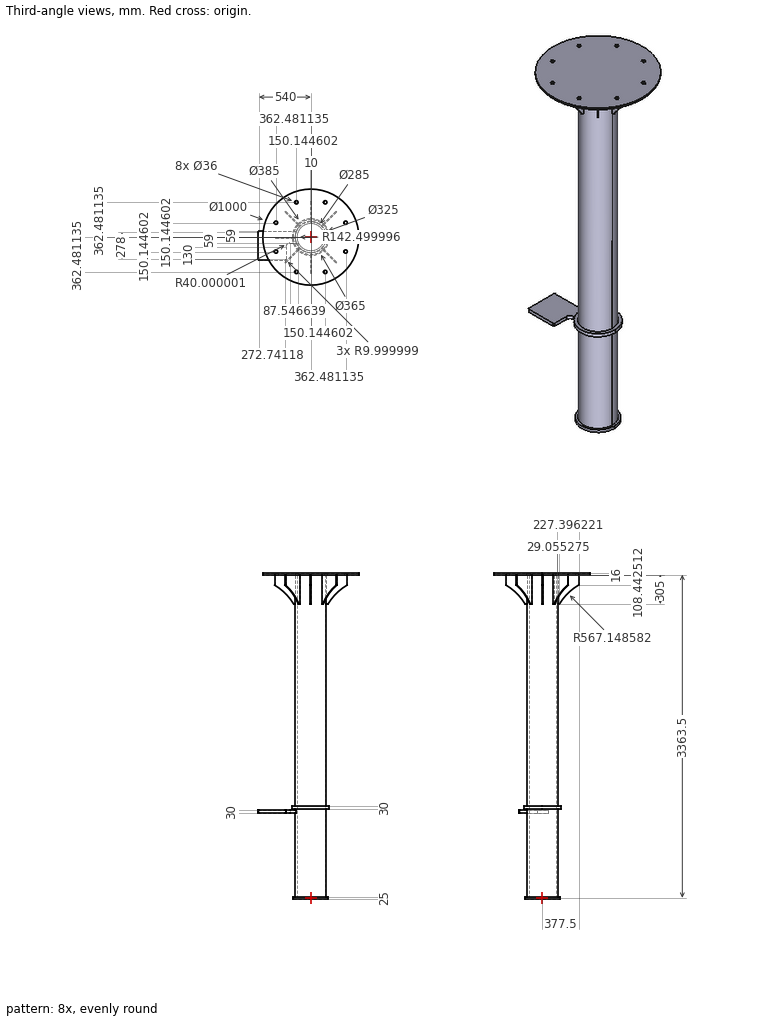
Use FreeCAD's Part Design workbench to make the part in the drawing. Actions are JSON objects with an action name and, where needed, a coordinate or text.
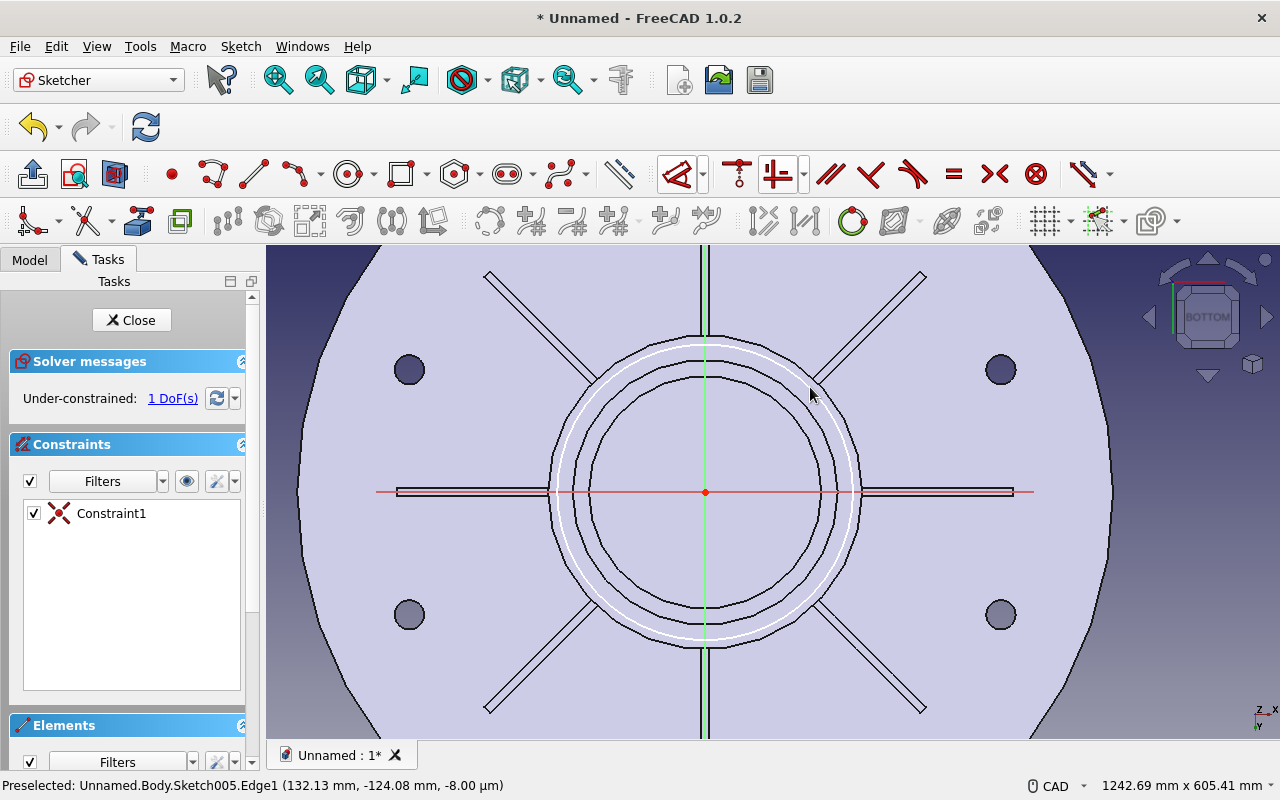
{"action": "left_click", "coordinate": [809, 387]}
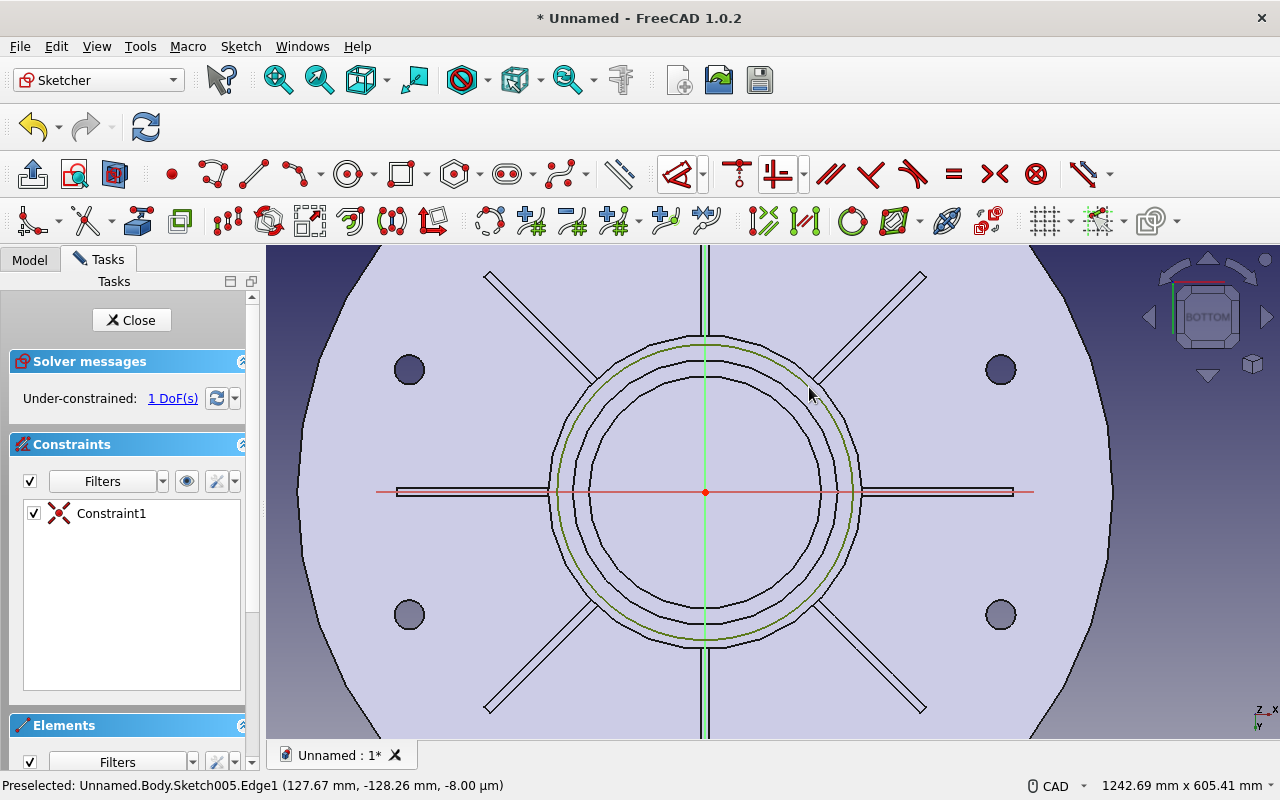
{"action": "left_click", "coordinate": [702, 174]}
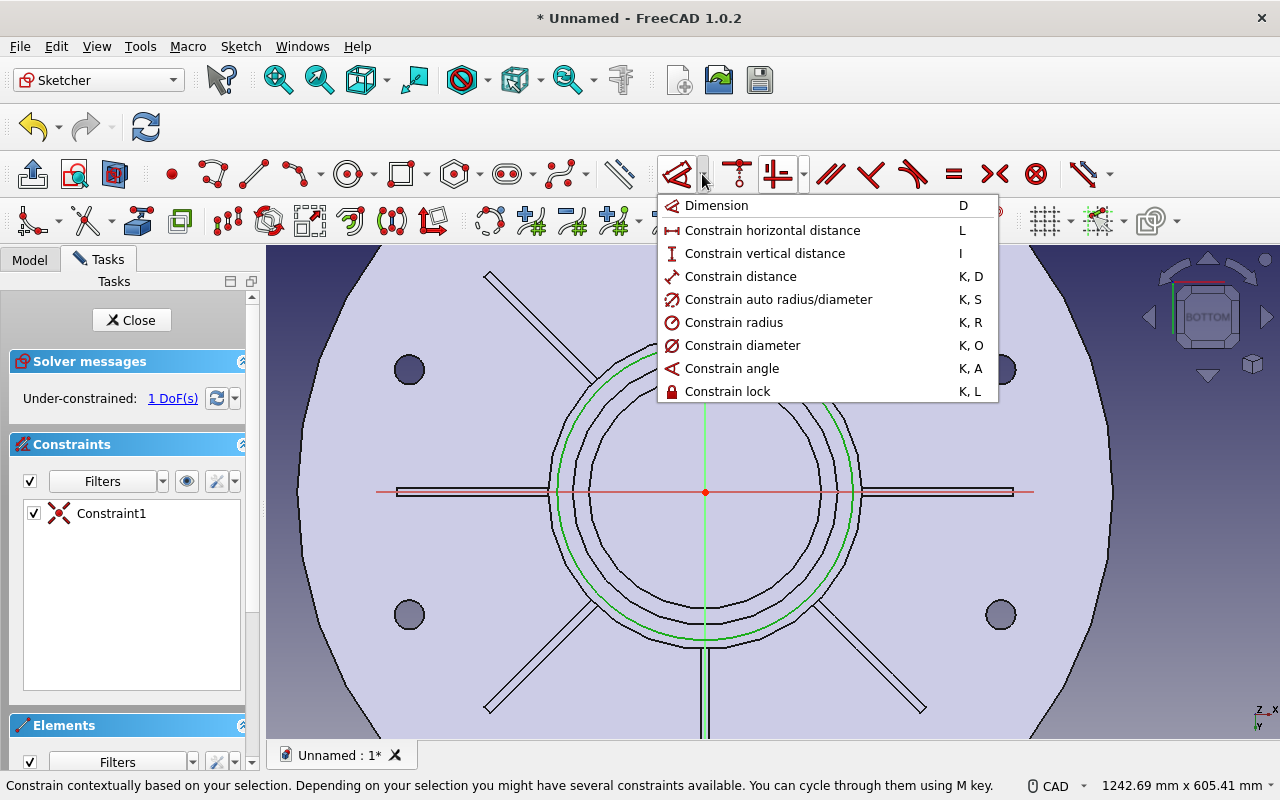
{"action": "left_click", "coordinate": [828, 346]}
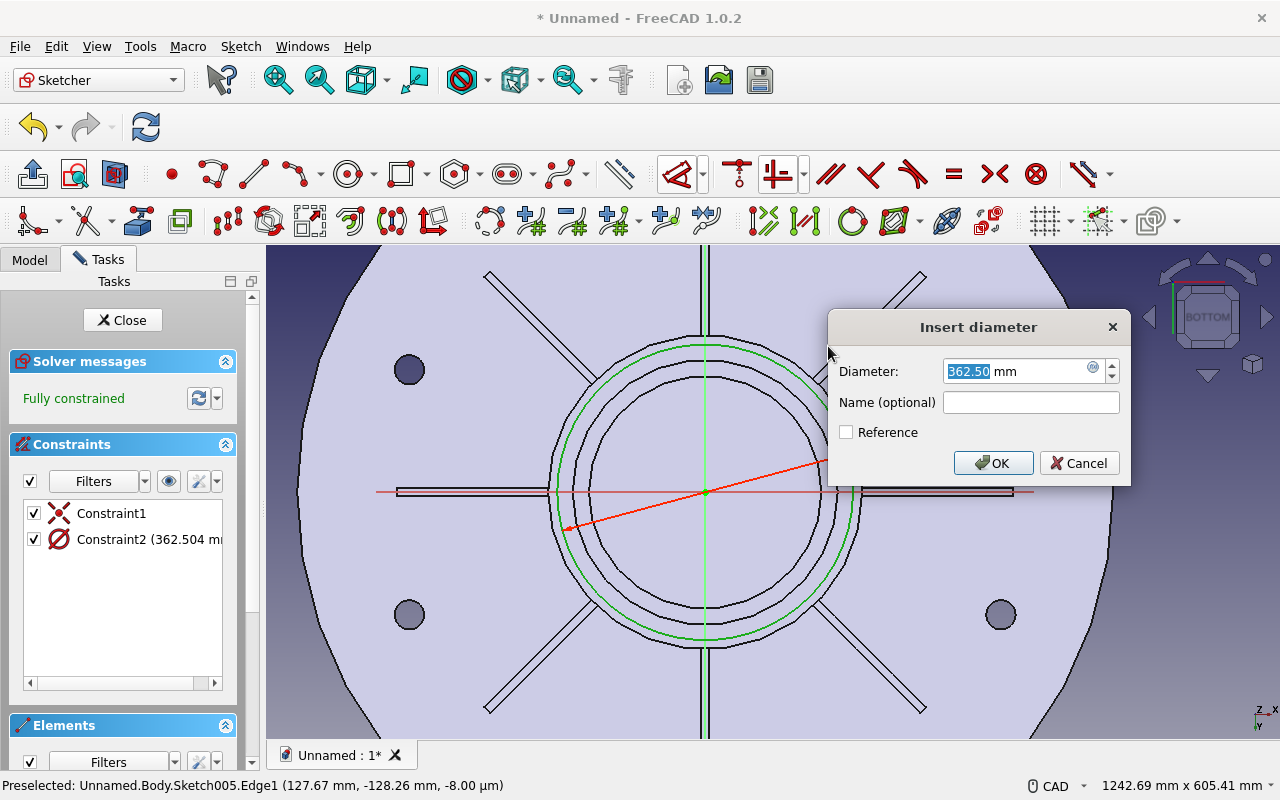
{"action": "type", "text": "365"}
{"action": "key", "text": "Return"}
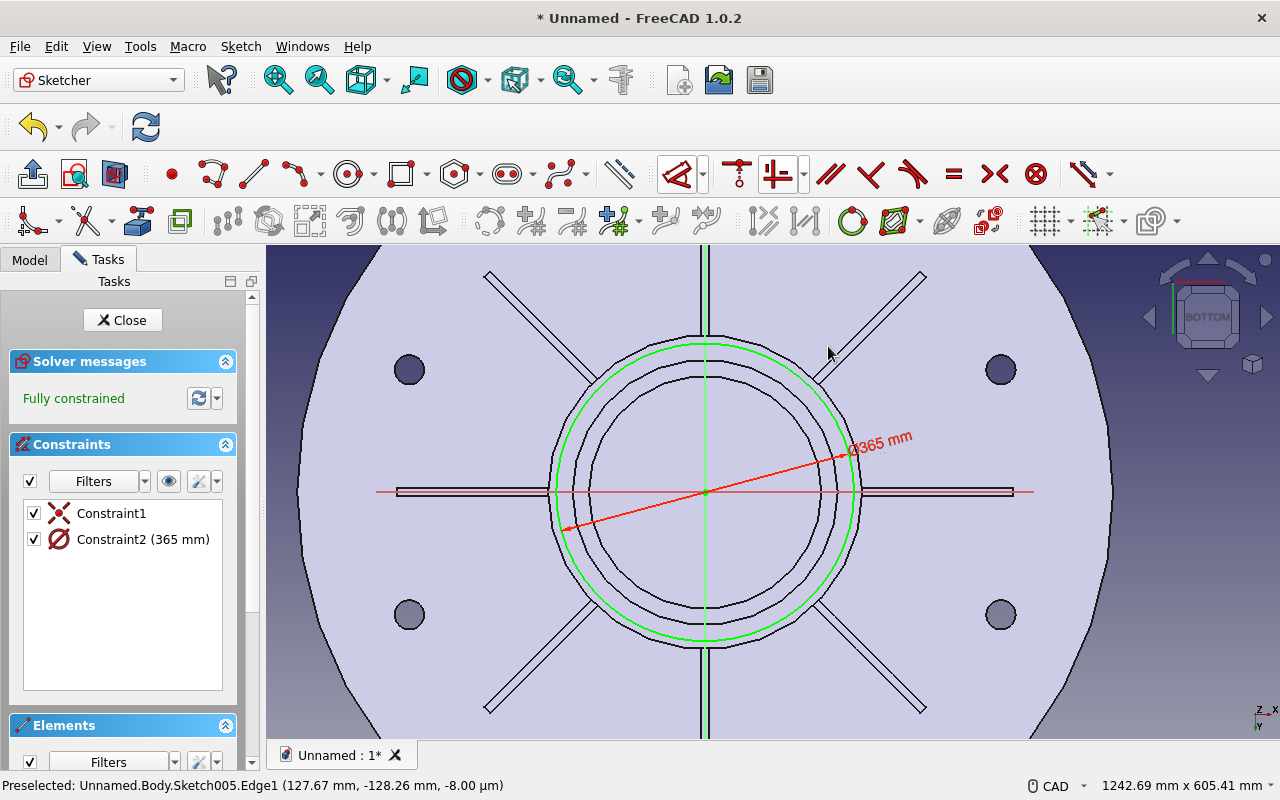
{"action": "left_click", "coordinate": [123, 320]}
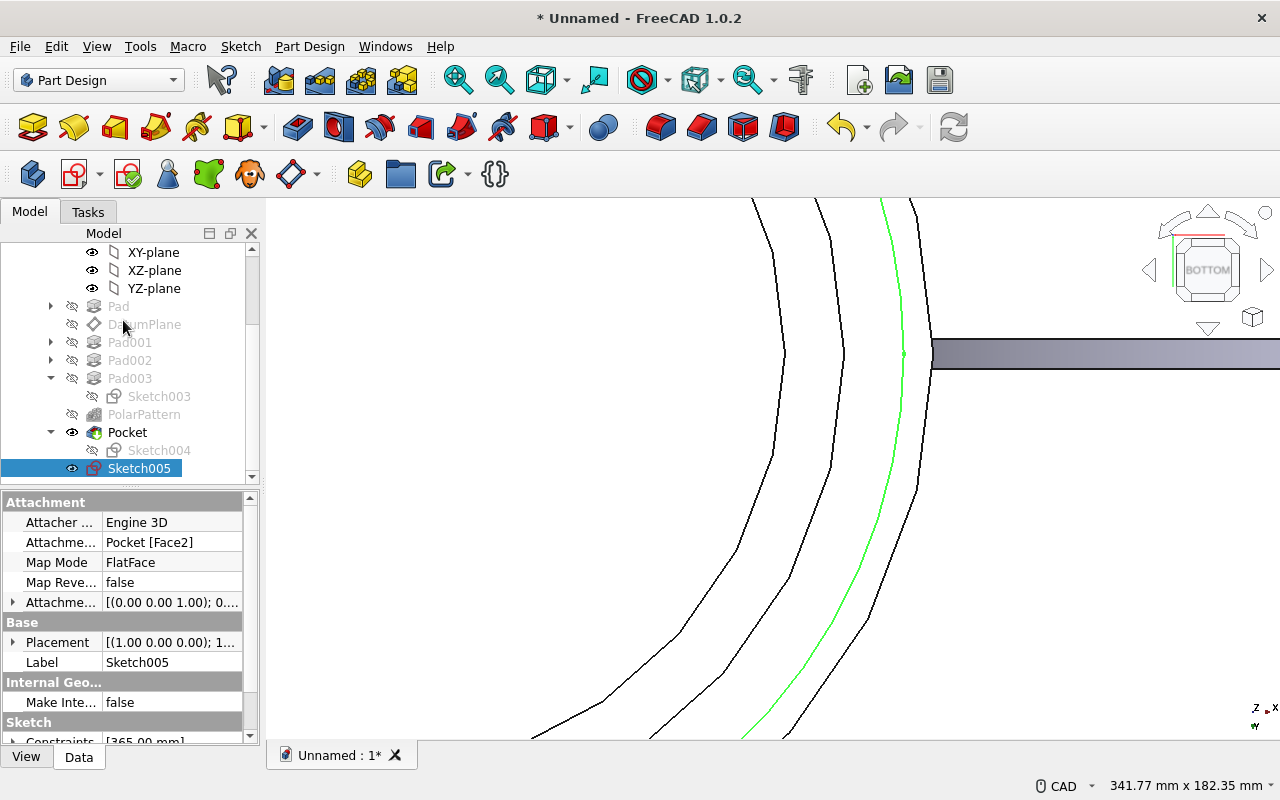
{"action": "left_click", "coordinate": [33, 128]}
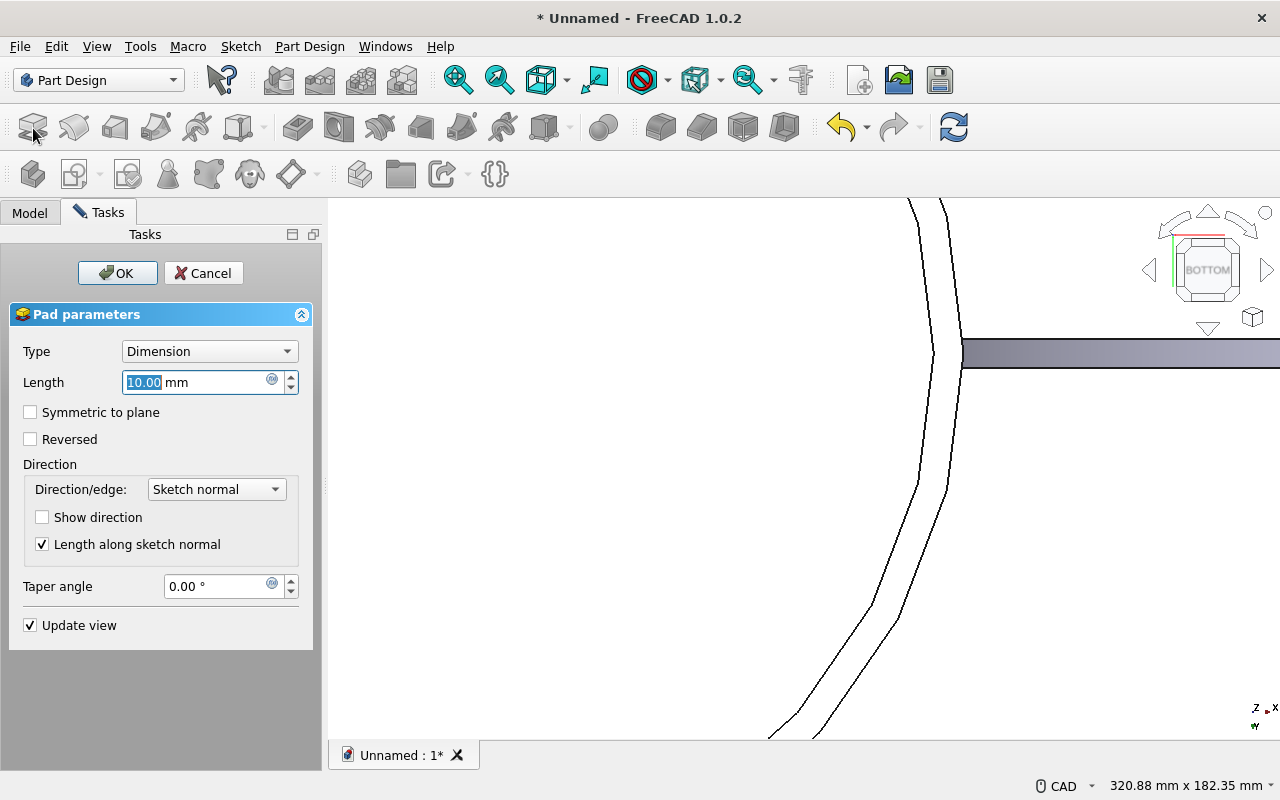
{"action": "type", "text": "25"}
{"action": "key", "text": "Tab"}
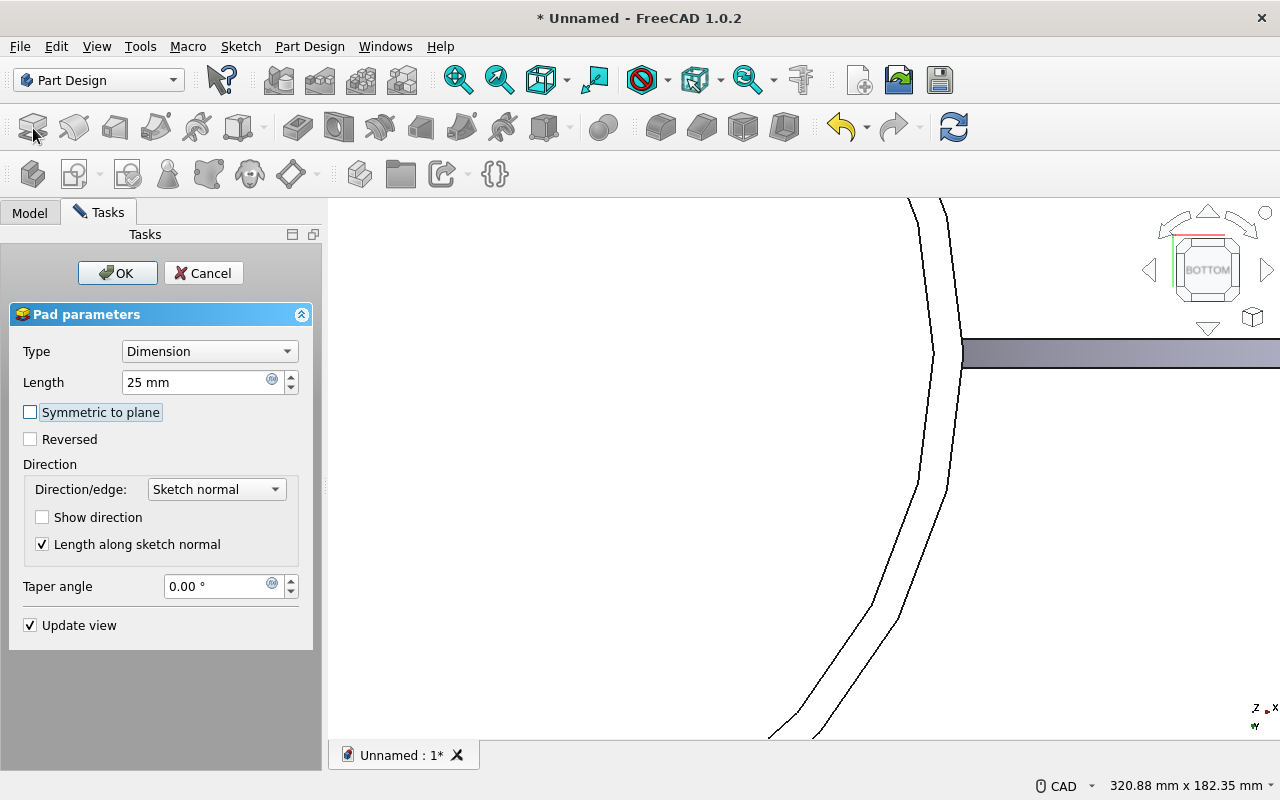
{"action": "left_click", "coordinate": [31, 412]}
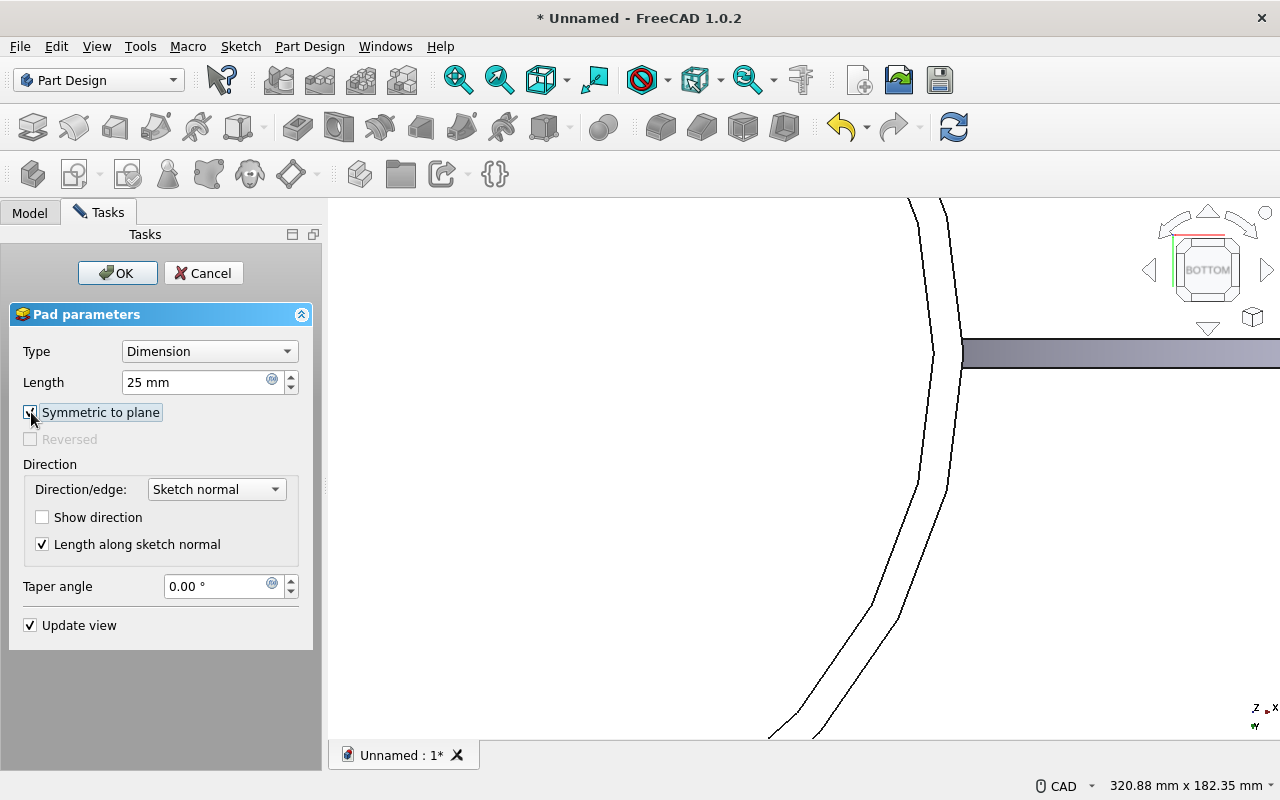
{"action": "left_click", "coordinate": [118, 273]}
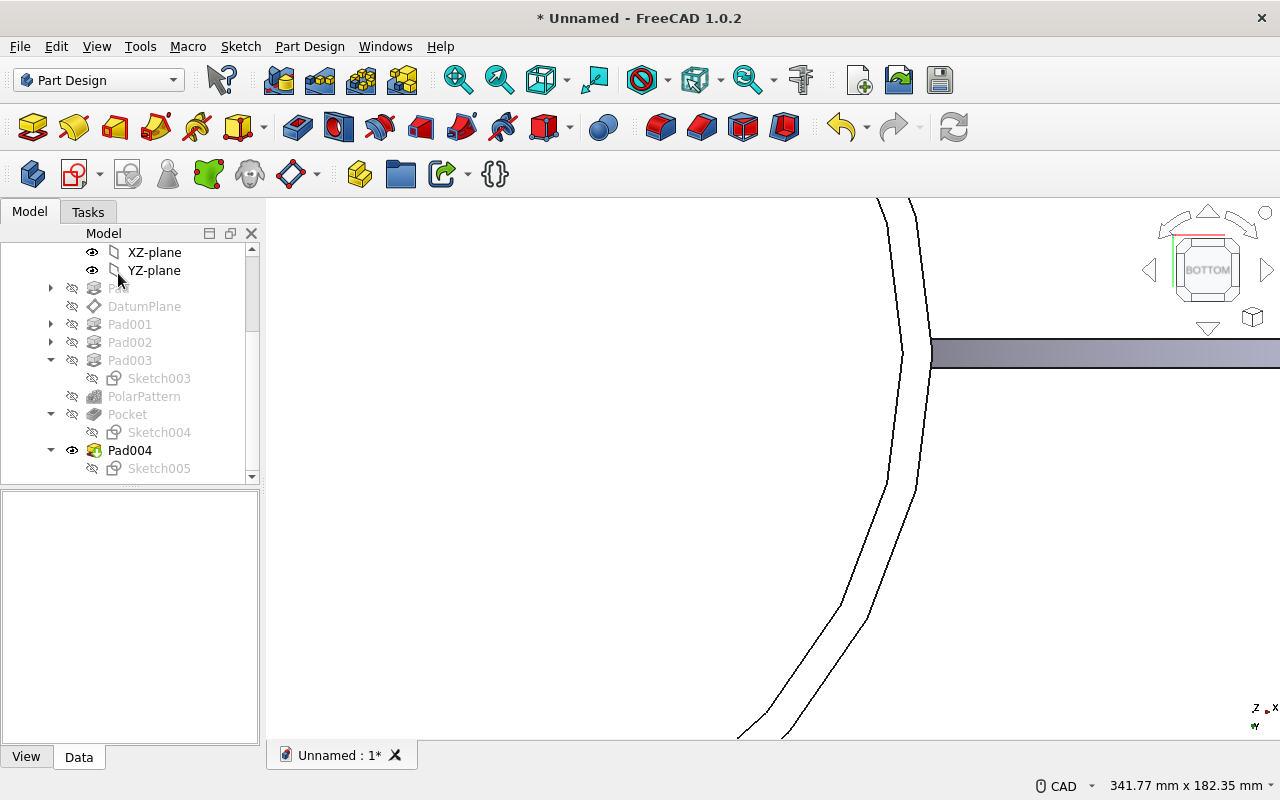
{"action": "key", "text": "v f"}